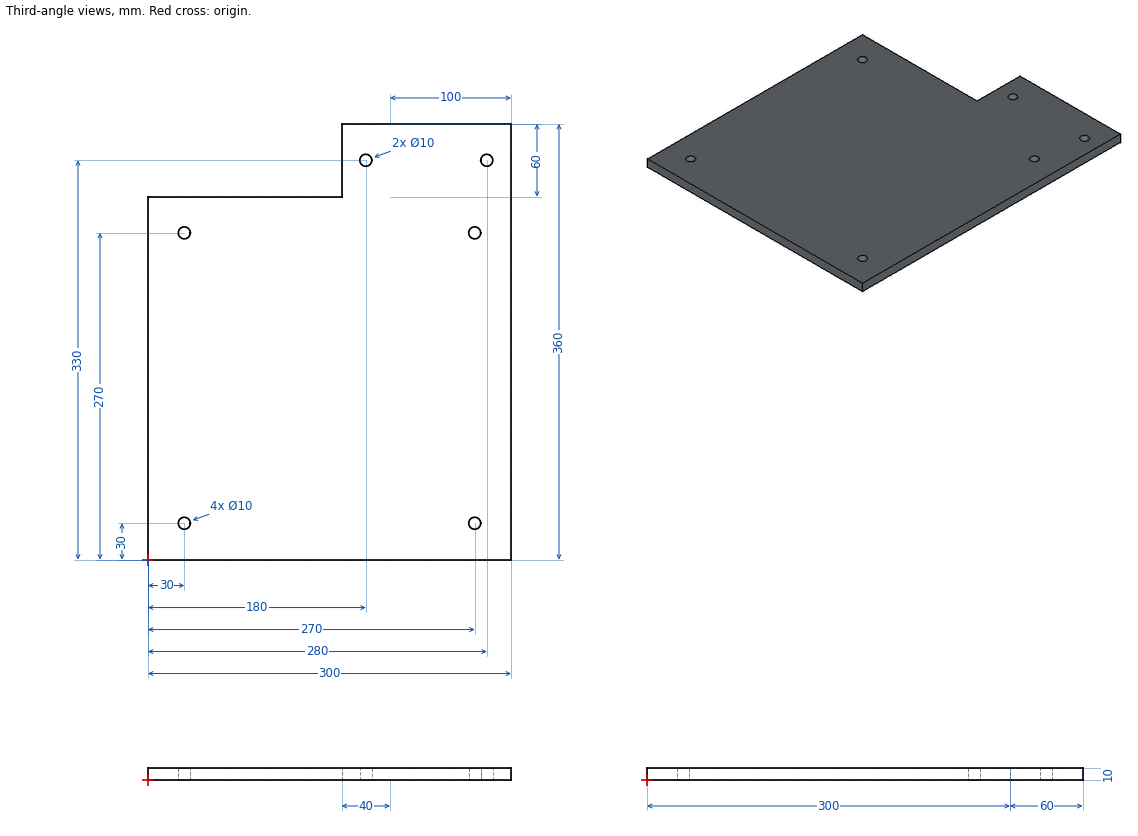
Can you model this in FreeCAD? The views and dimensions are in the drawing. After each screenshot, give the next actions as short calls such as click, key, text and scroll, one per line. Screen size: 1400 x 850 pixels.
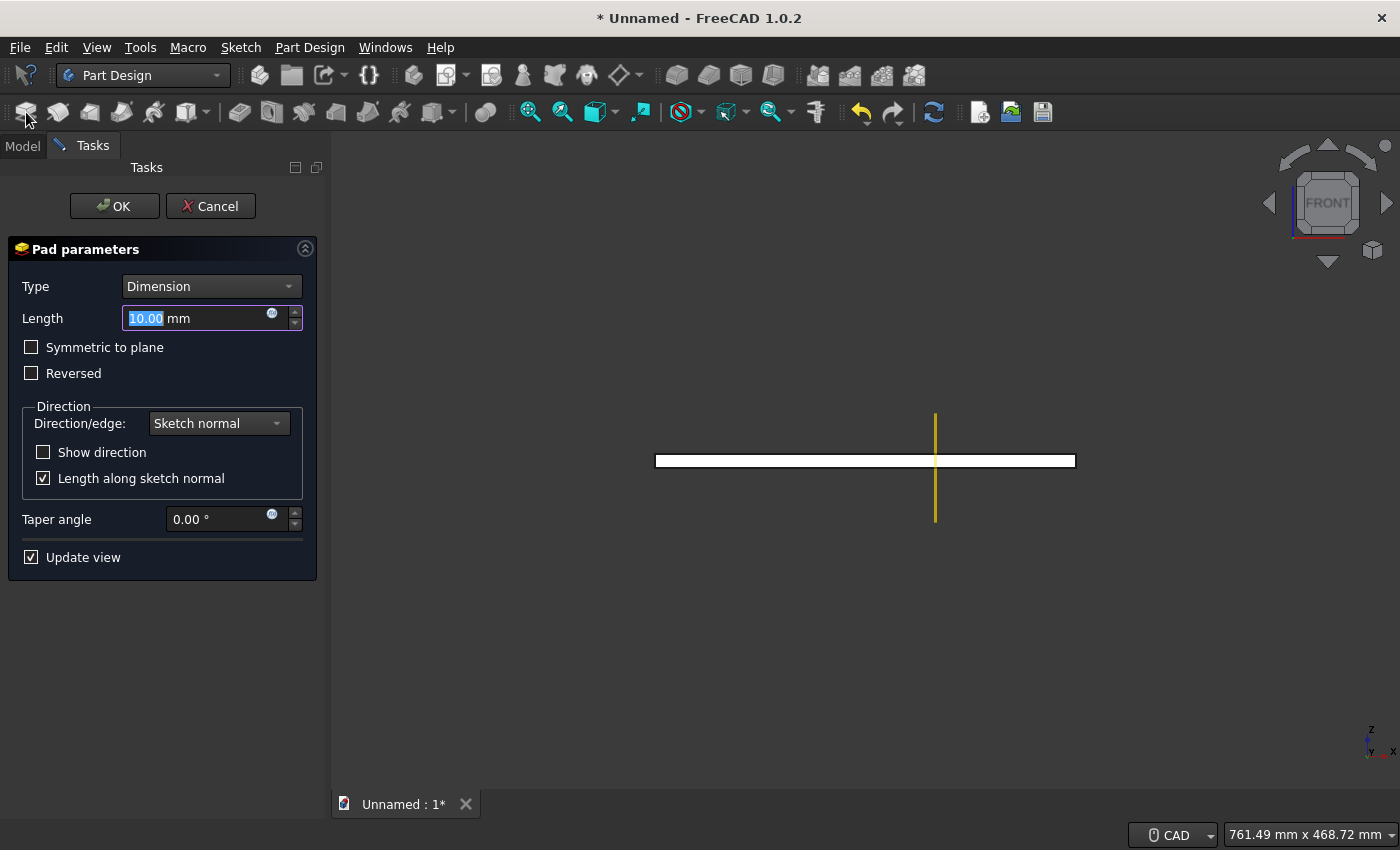
text(40)
key(Tab)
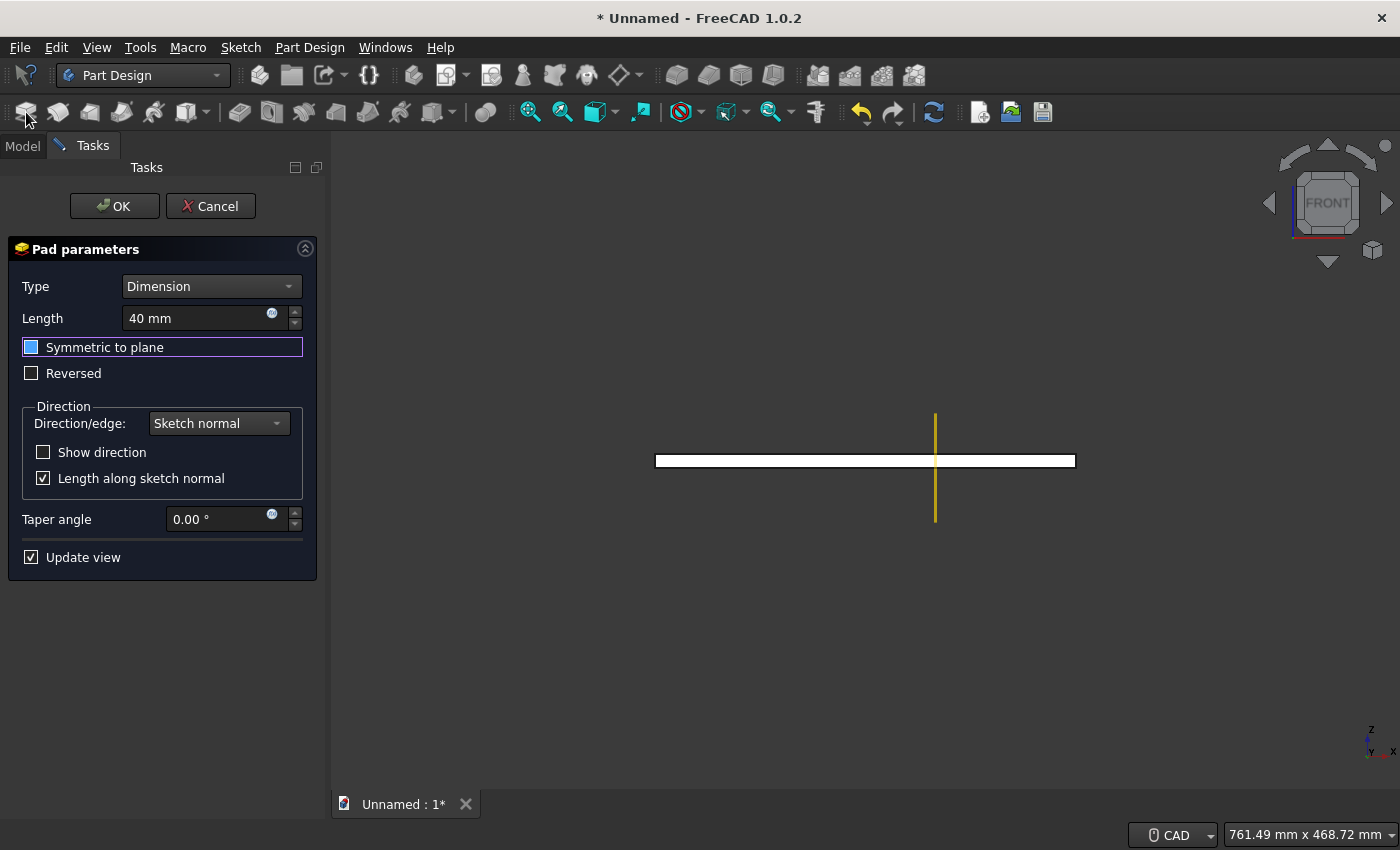
click(30, 373)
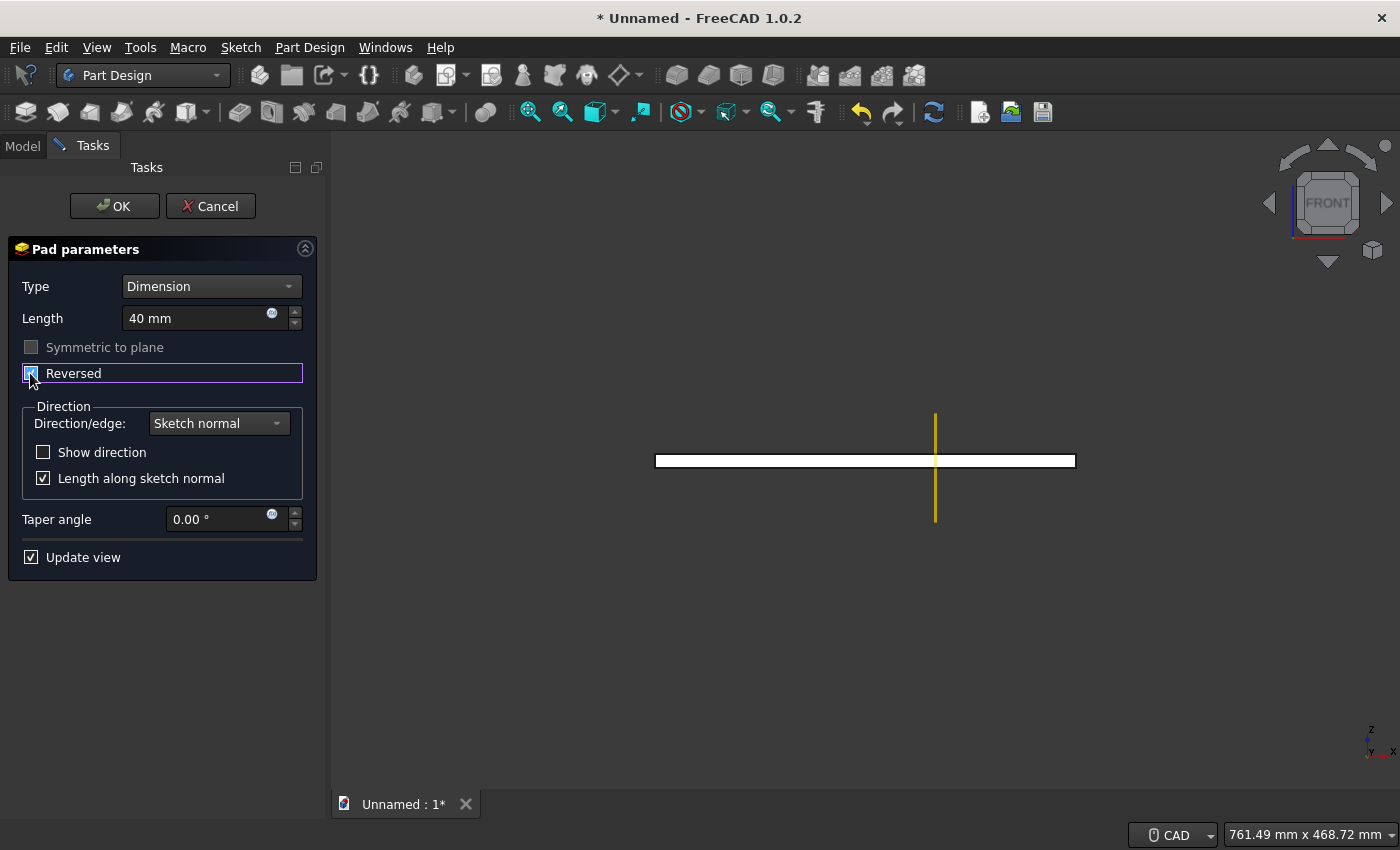
click(115, 206)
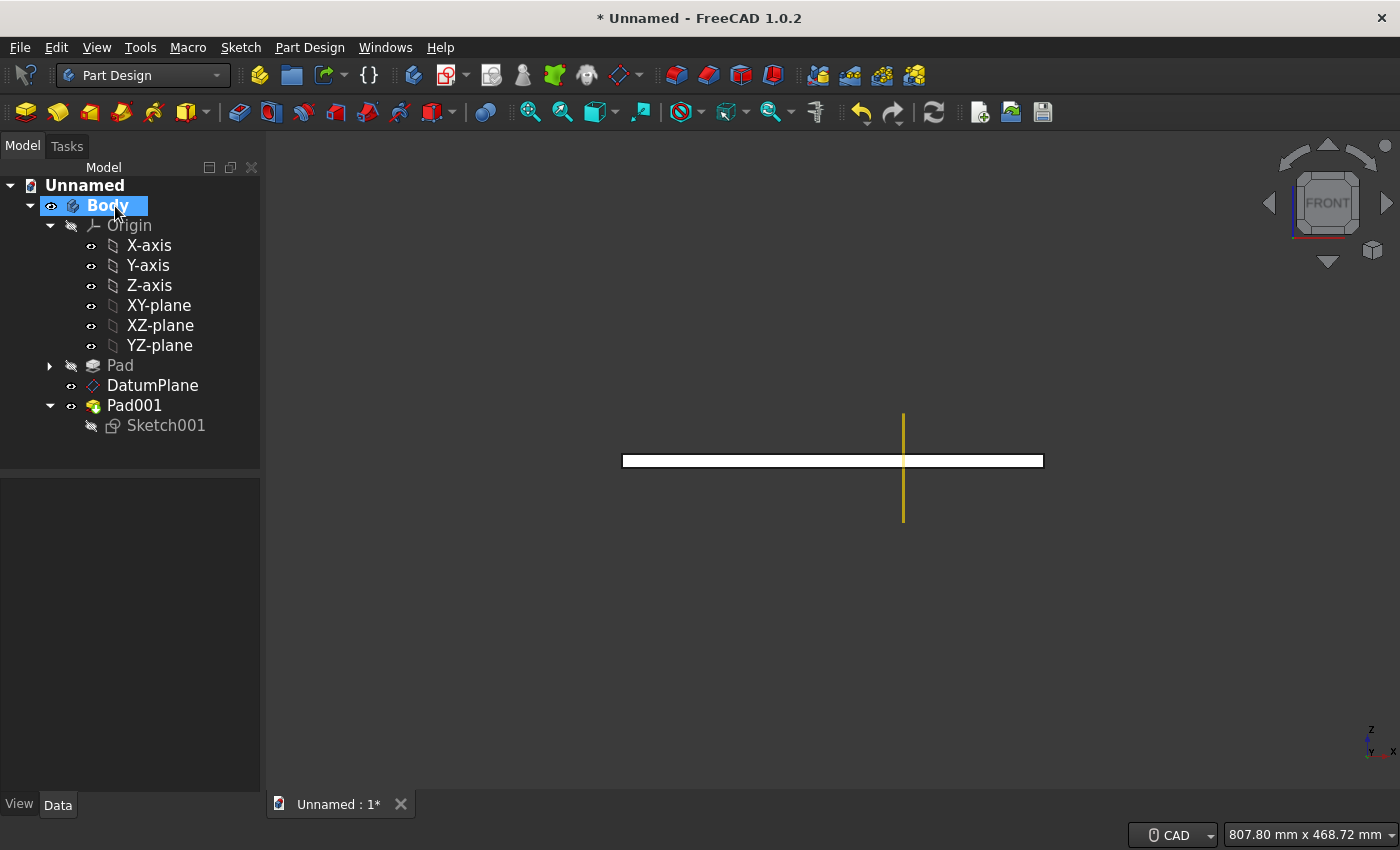
click(116, 386)
key(space)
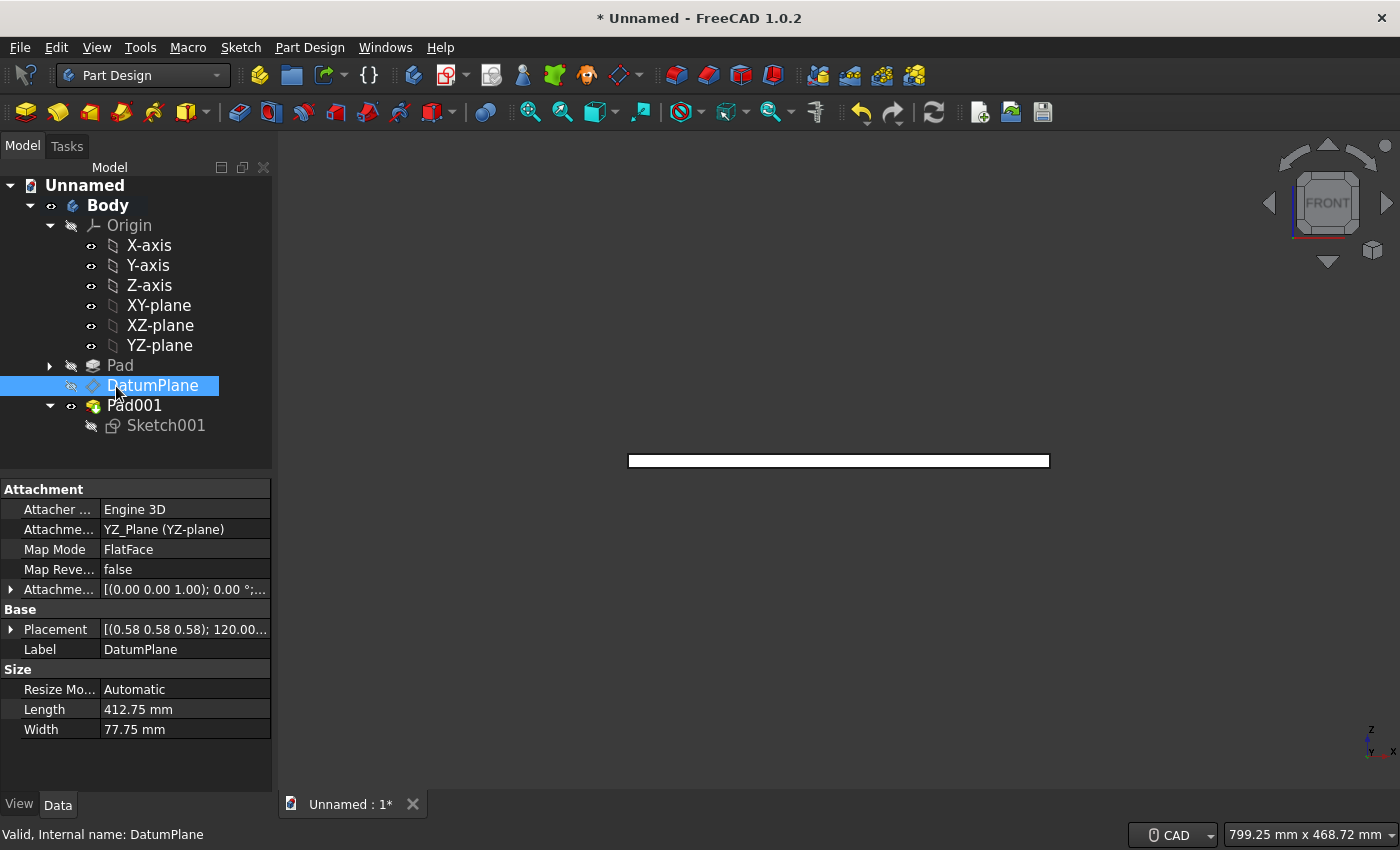
click(532, 112)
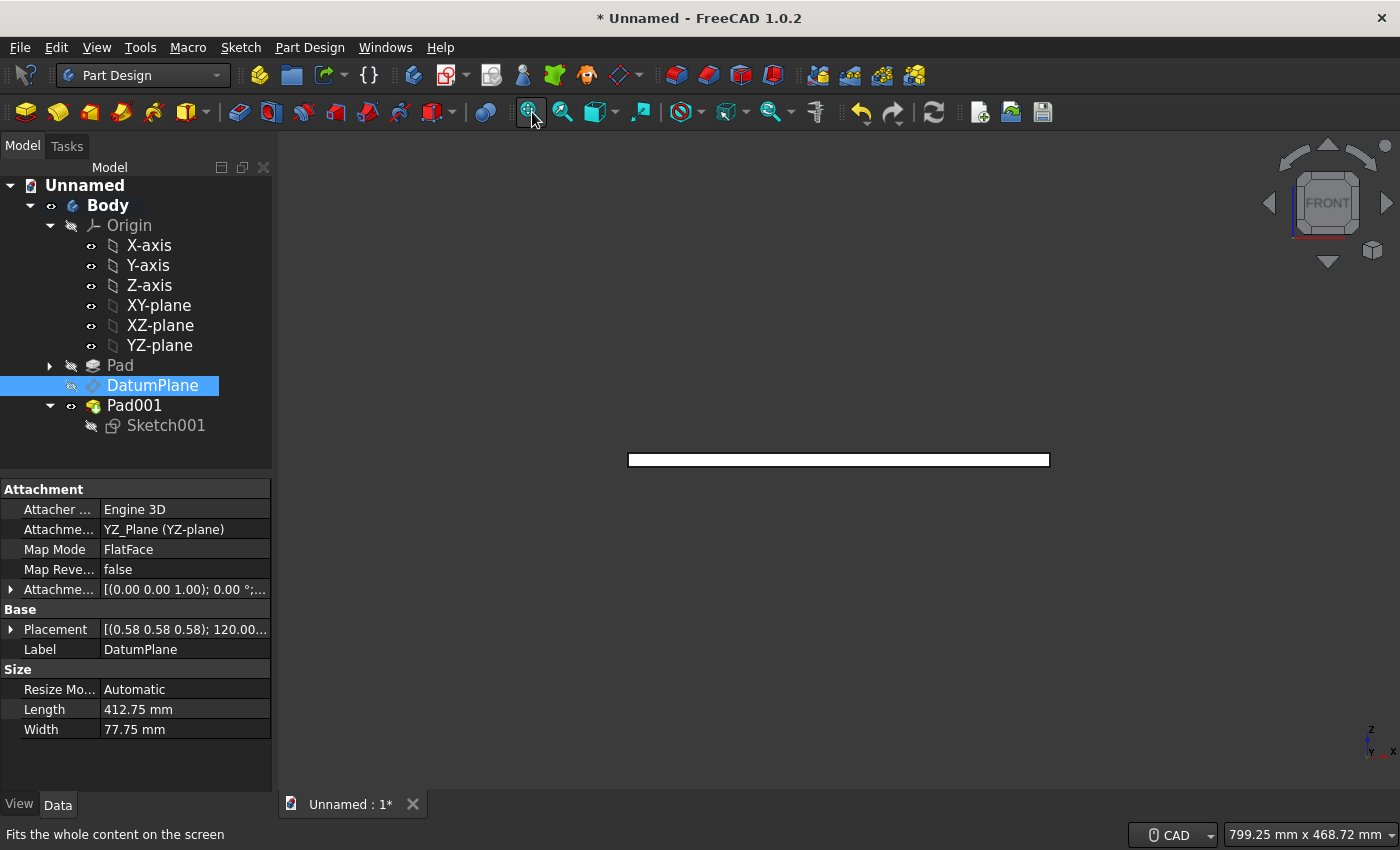
key(0)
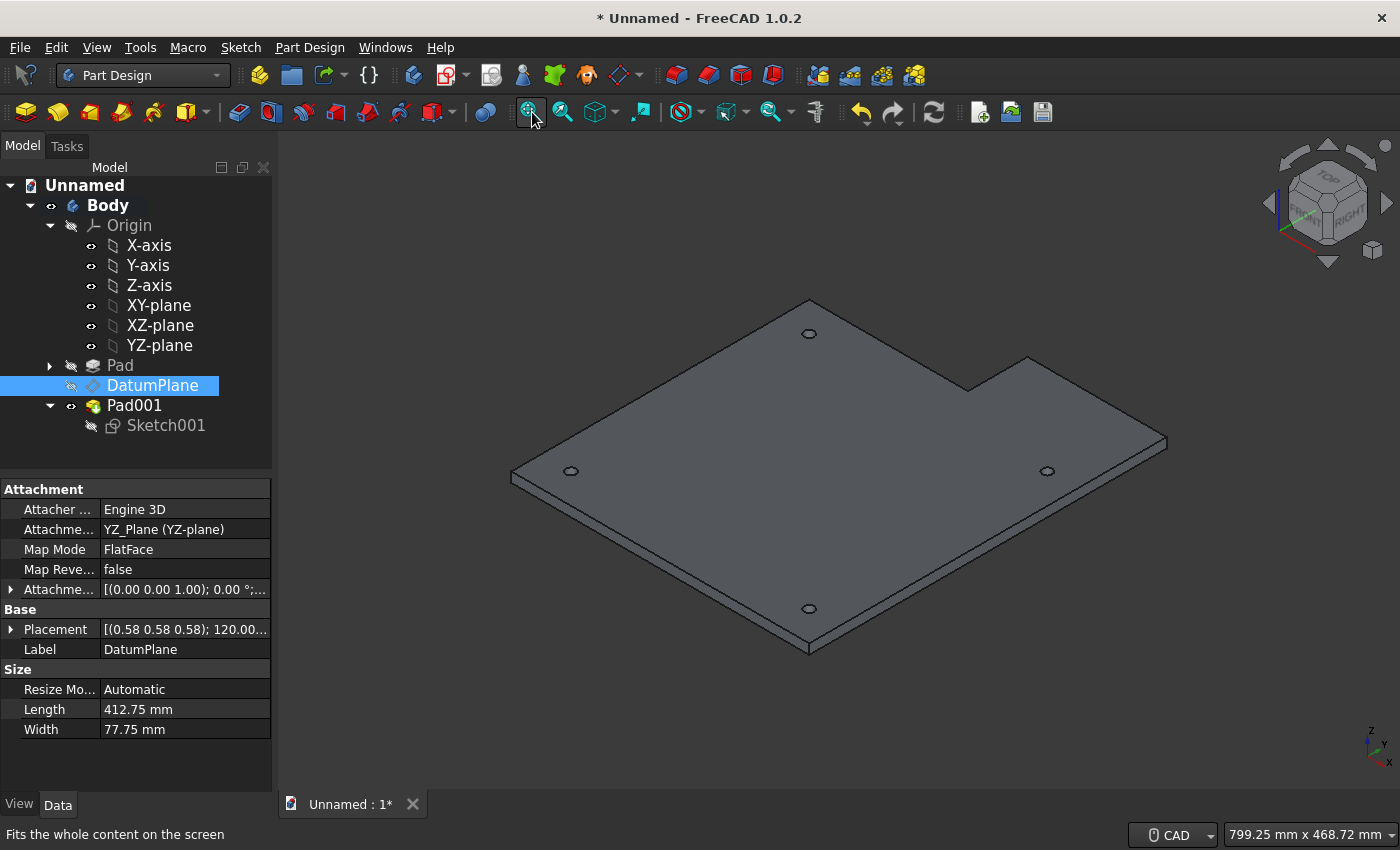
click(788, 483)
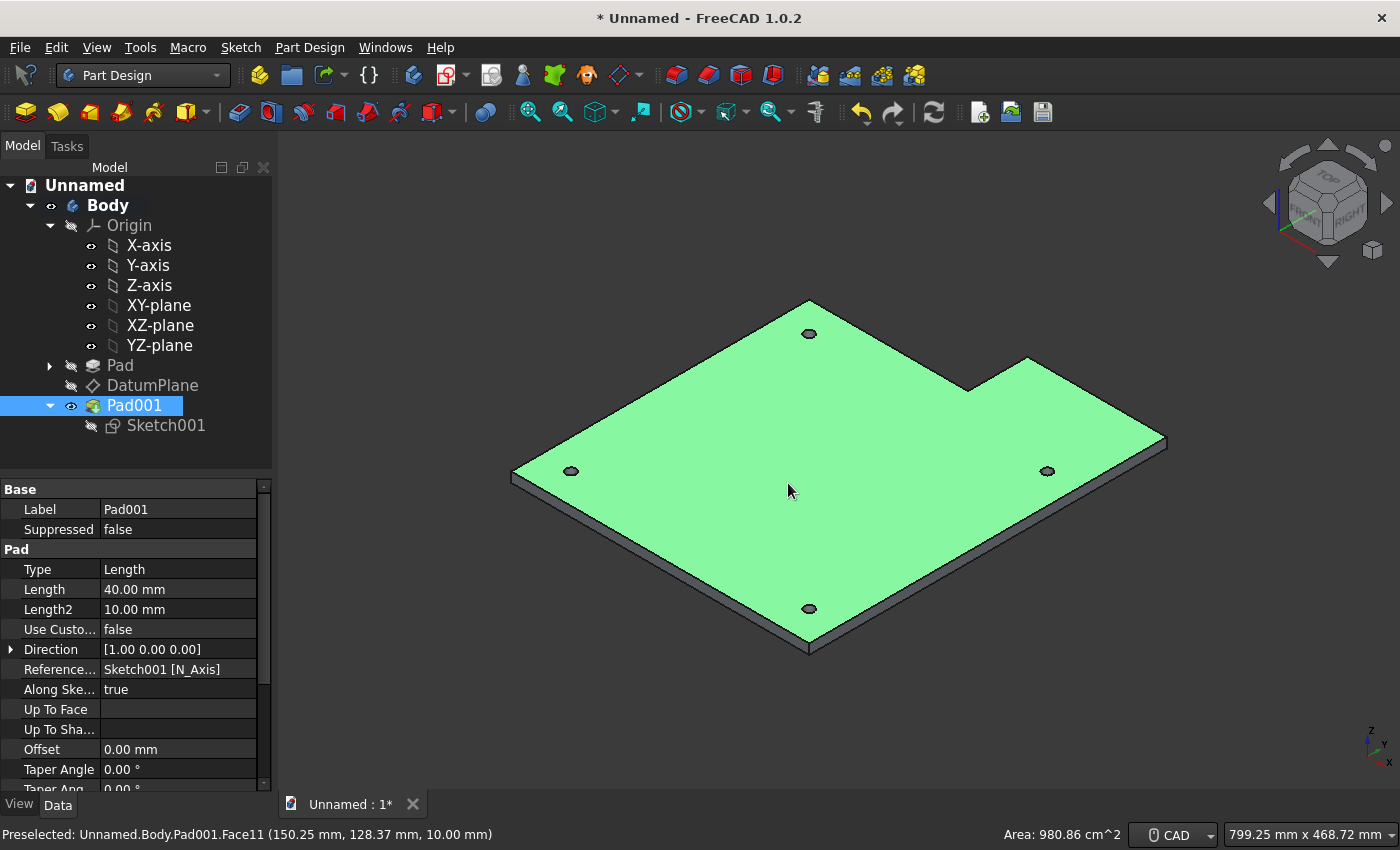
click(446, 76)